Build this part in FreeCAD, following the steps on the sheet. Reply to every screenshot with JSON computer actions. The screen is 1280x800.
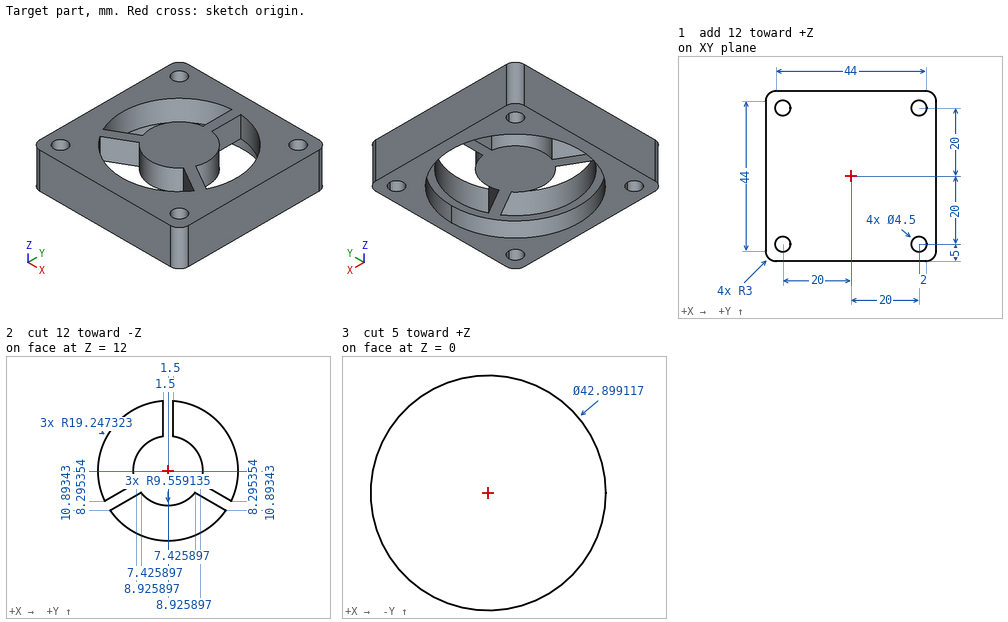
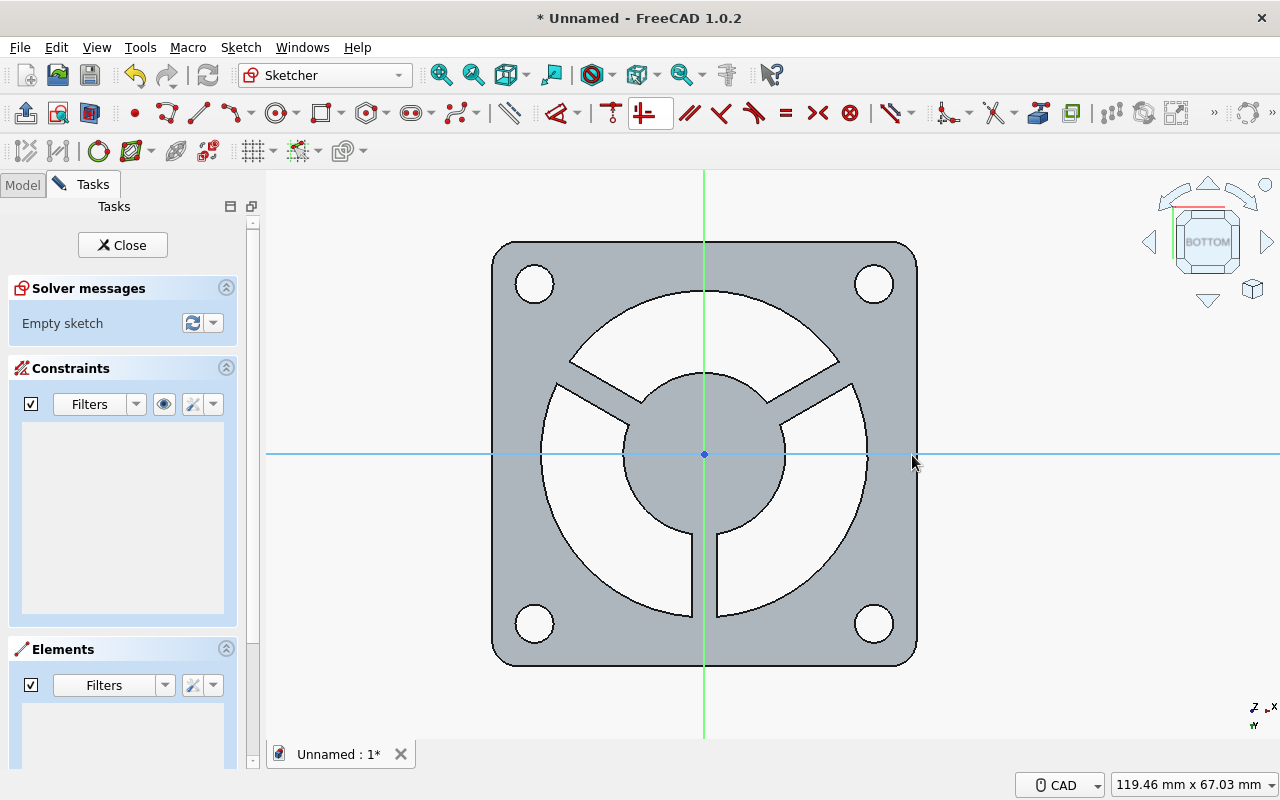
{"action": "left_click", "coordinate": [276, 114]}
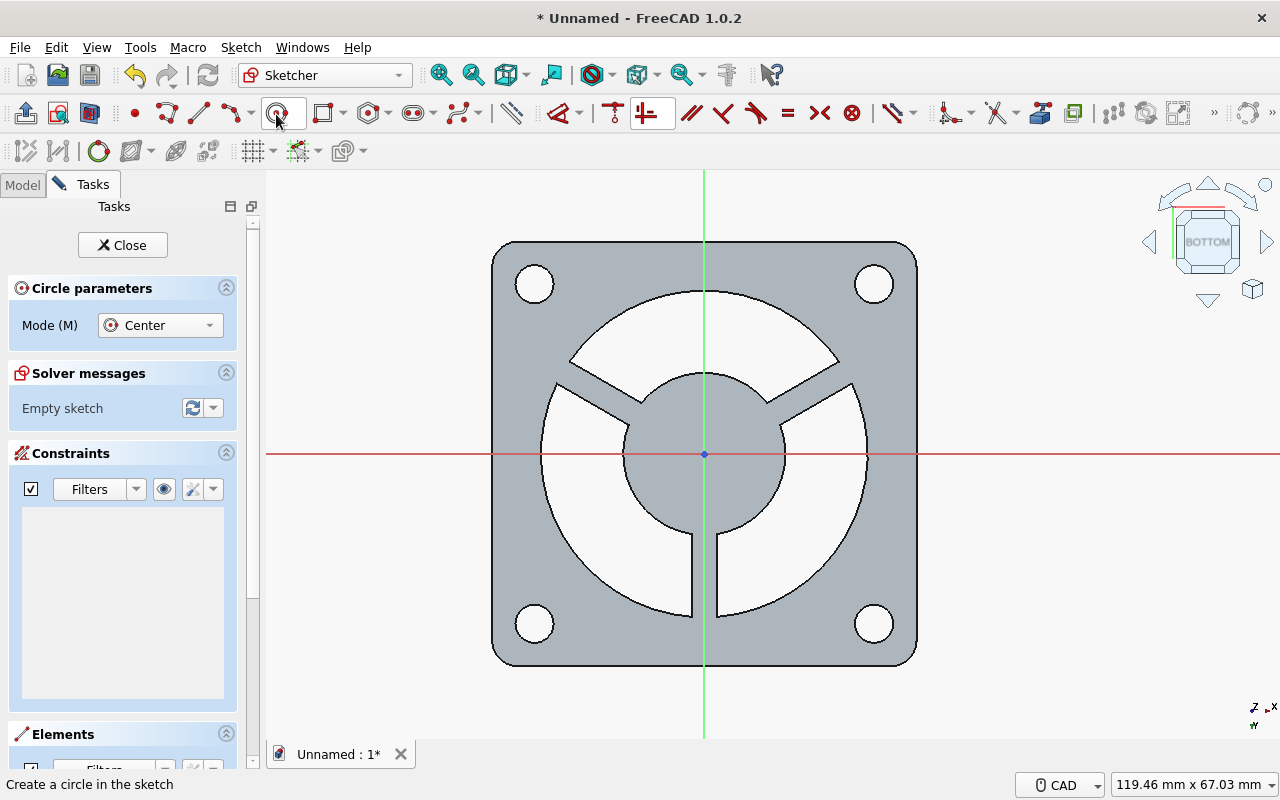
{"action": "left_click", "coordinate": [704, 454]}
{"action": "left_click", "coordinate": [833, 325]}
{"action": "key", "text": "Escape"}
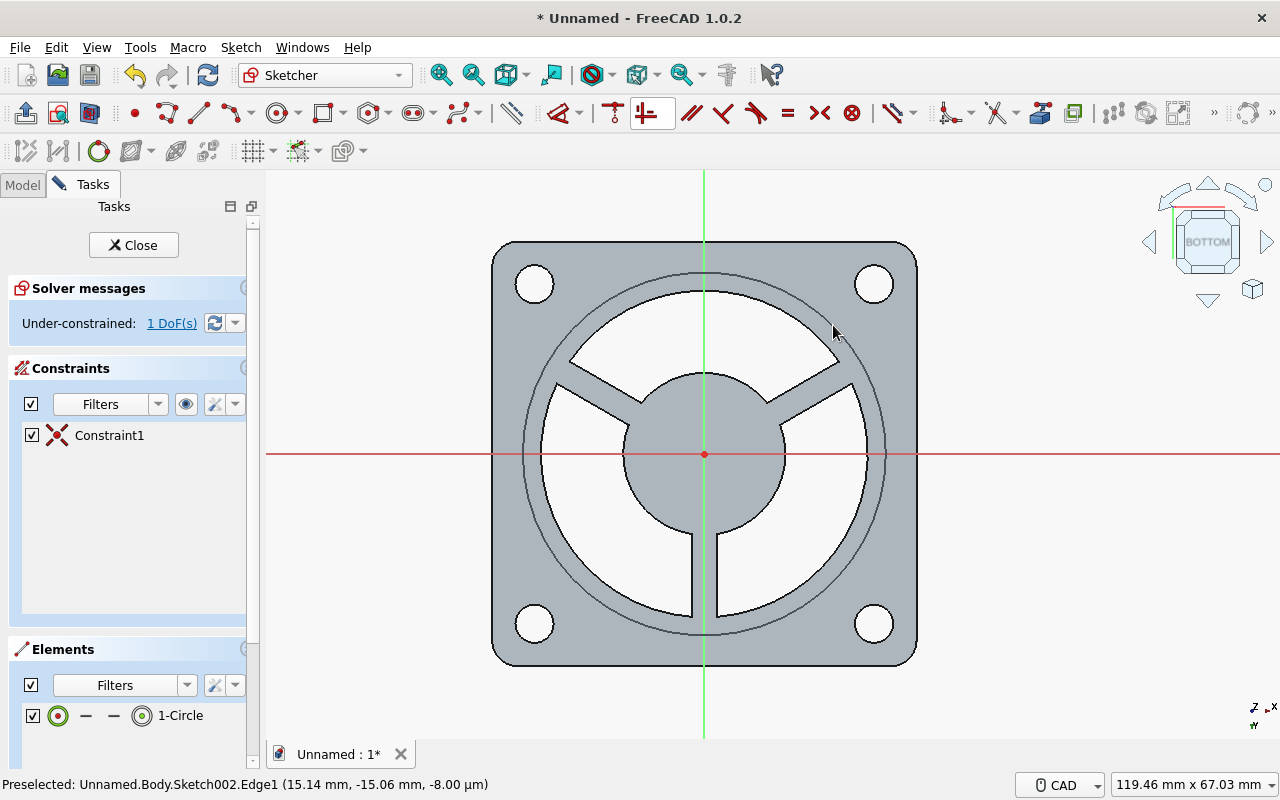
{"action": "left_click", "coordinate": [558, 114]}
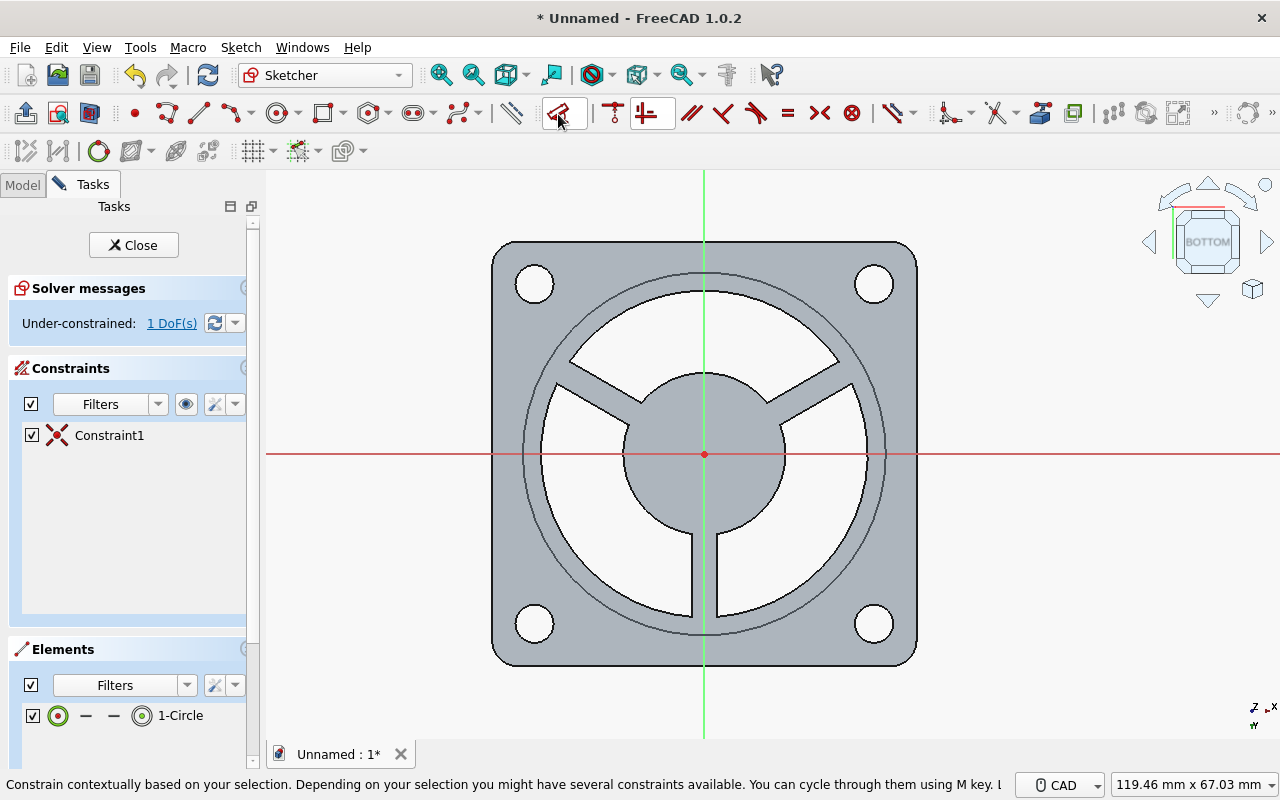
{"action": "left_click", "coordinate": [832, 325]}
{"action": "left_click", "coordinate": [855, 302]}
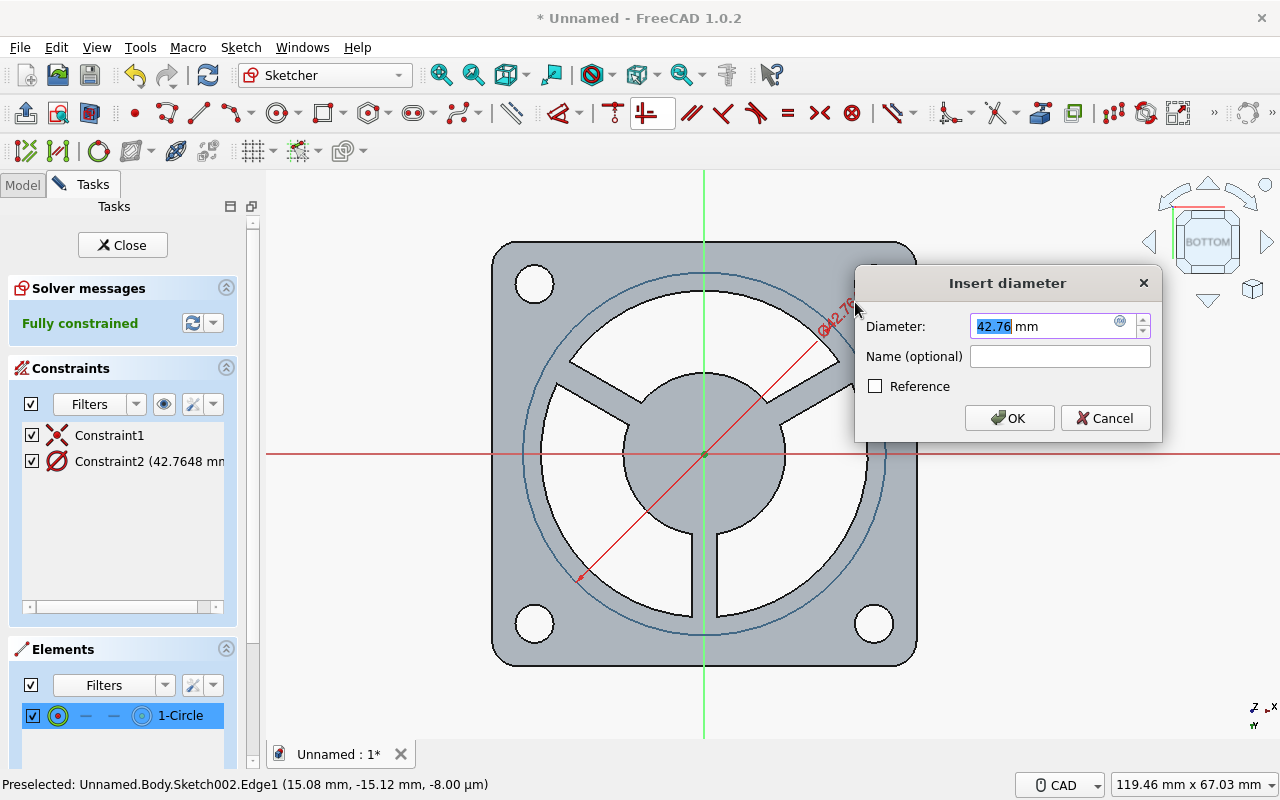
{"action": "type", "text": "42.899117"}
{"action": "key", "text": "Return"}
{"action": "key", "text": "Escape"}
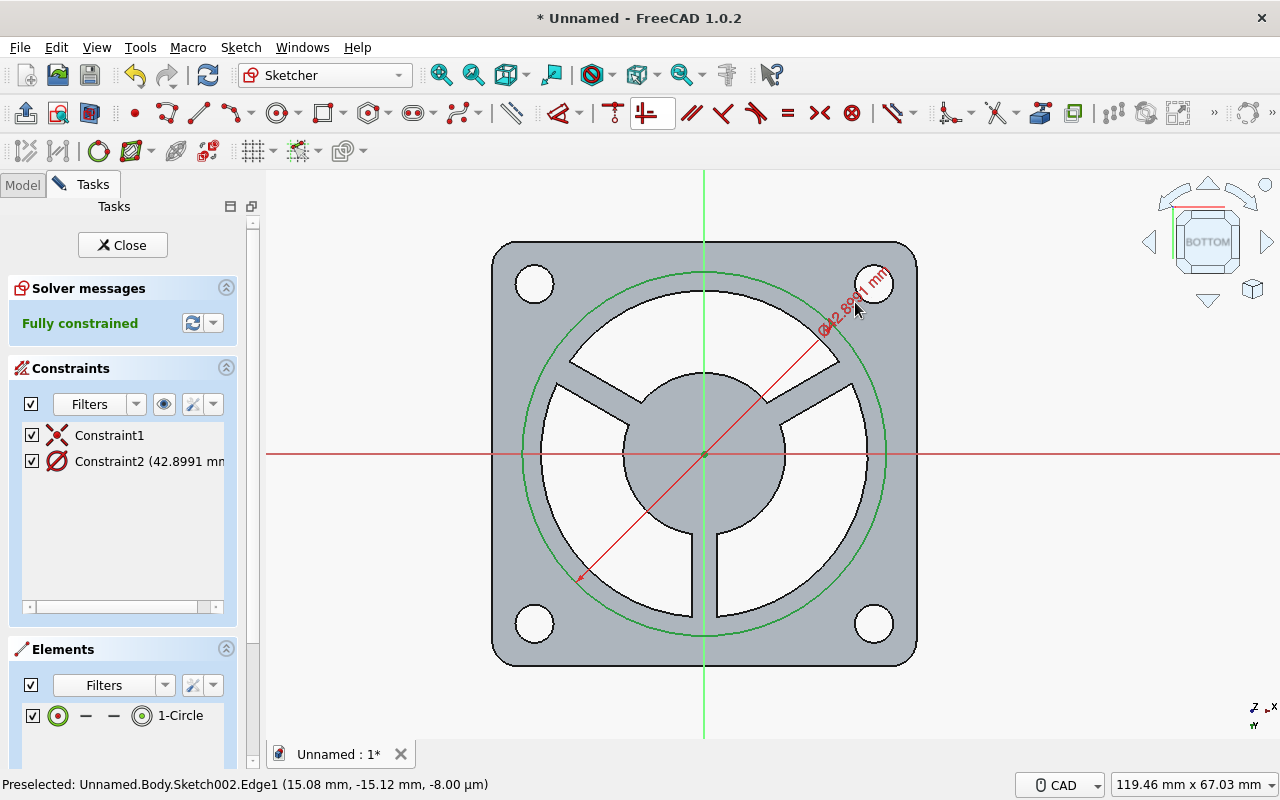
{"action": "left_click", "coordinate": [123, 245]}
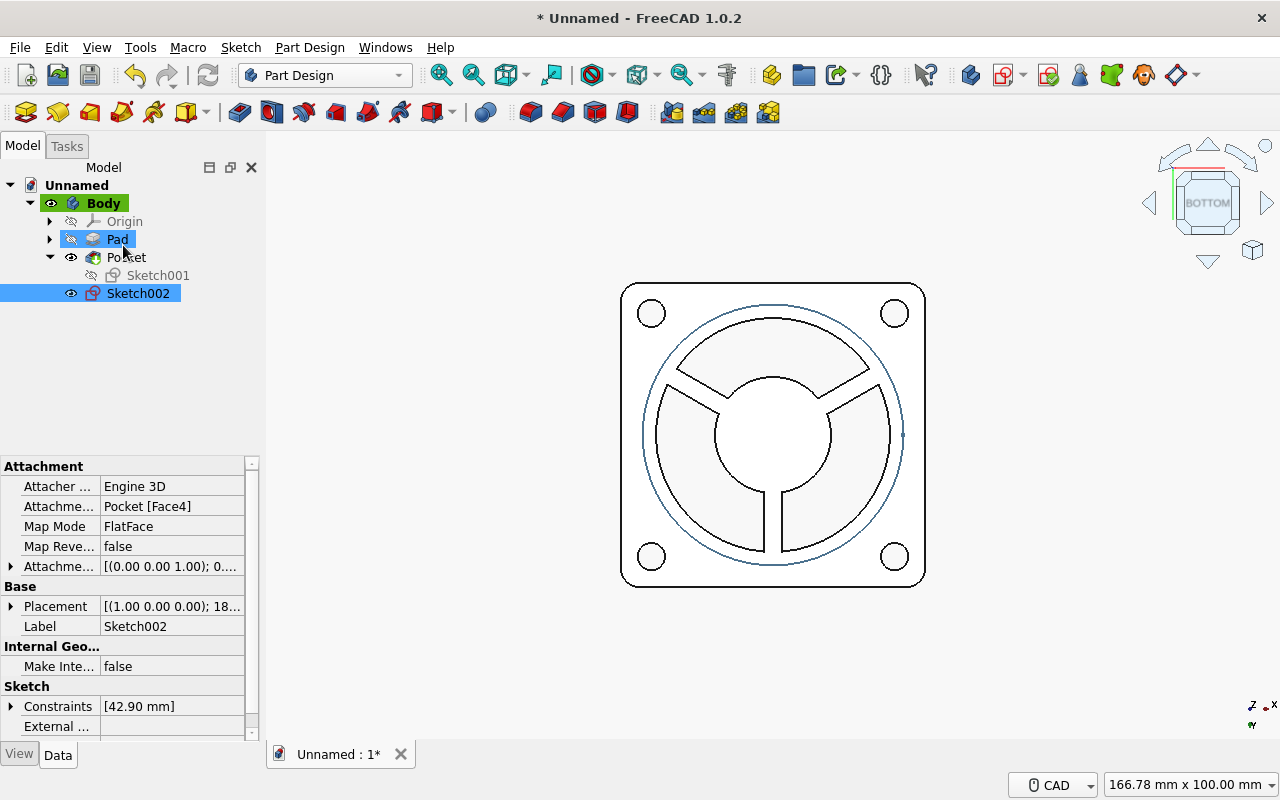
{"action": "left_click", "coordinate": [240, 112]}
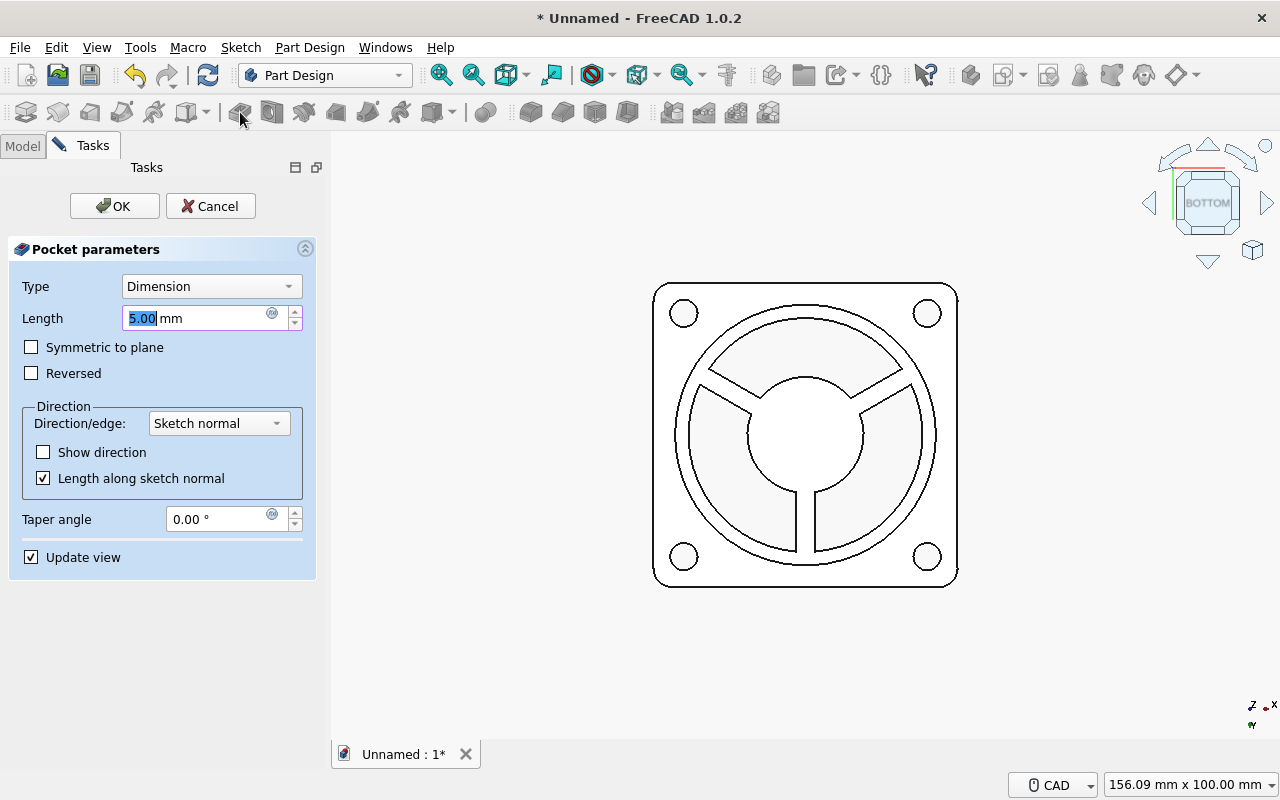
{"action": "type", "text": "5"}
{"action": "key", "text": "Tab"}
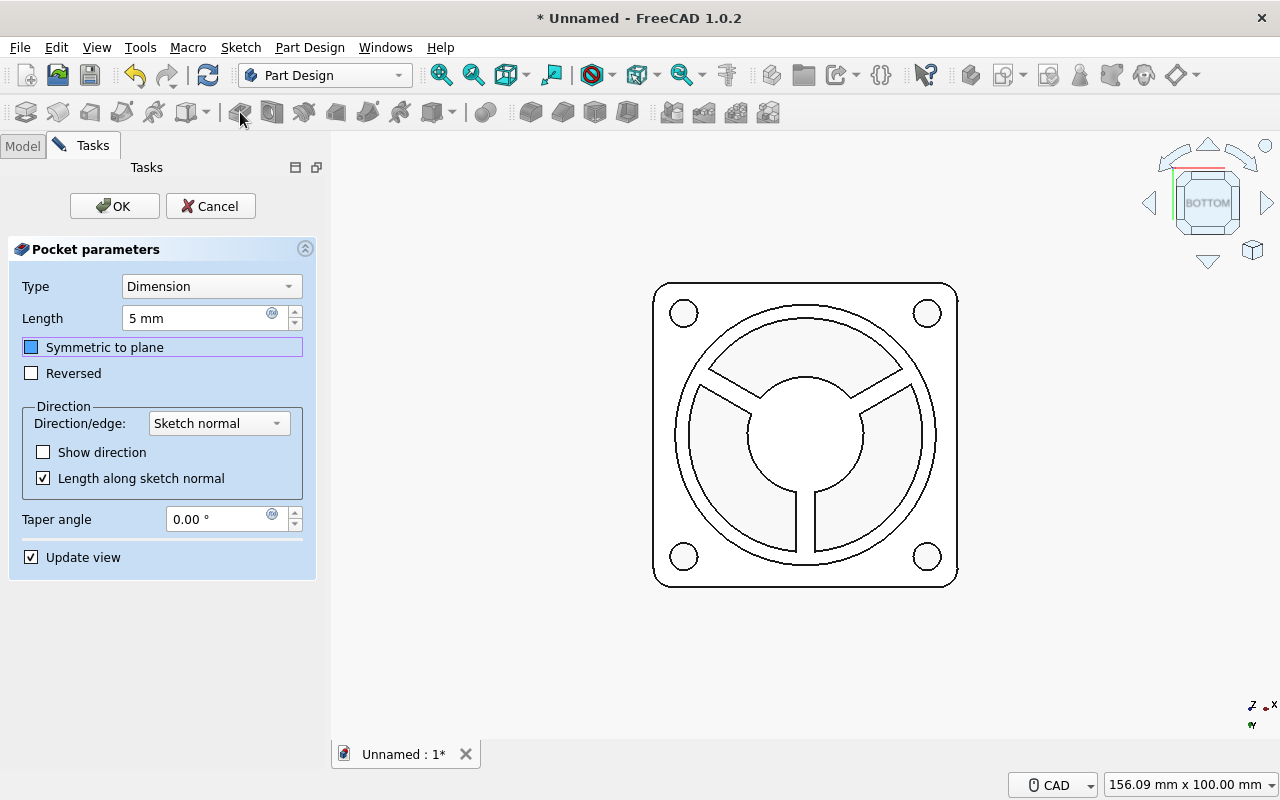
{"action": "left_click", "coordinate": [115, 206]}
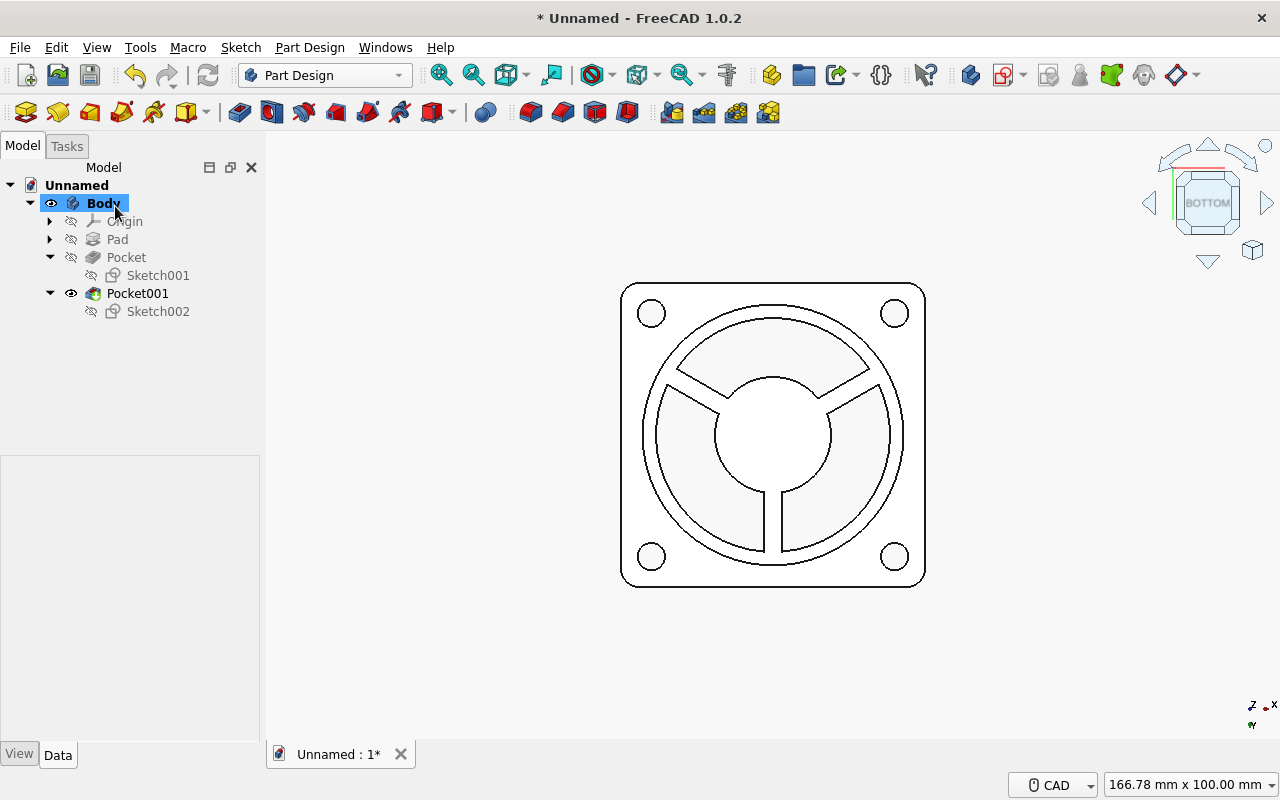
{"action": "key", "text": "0"}